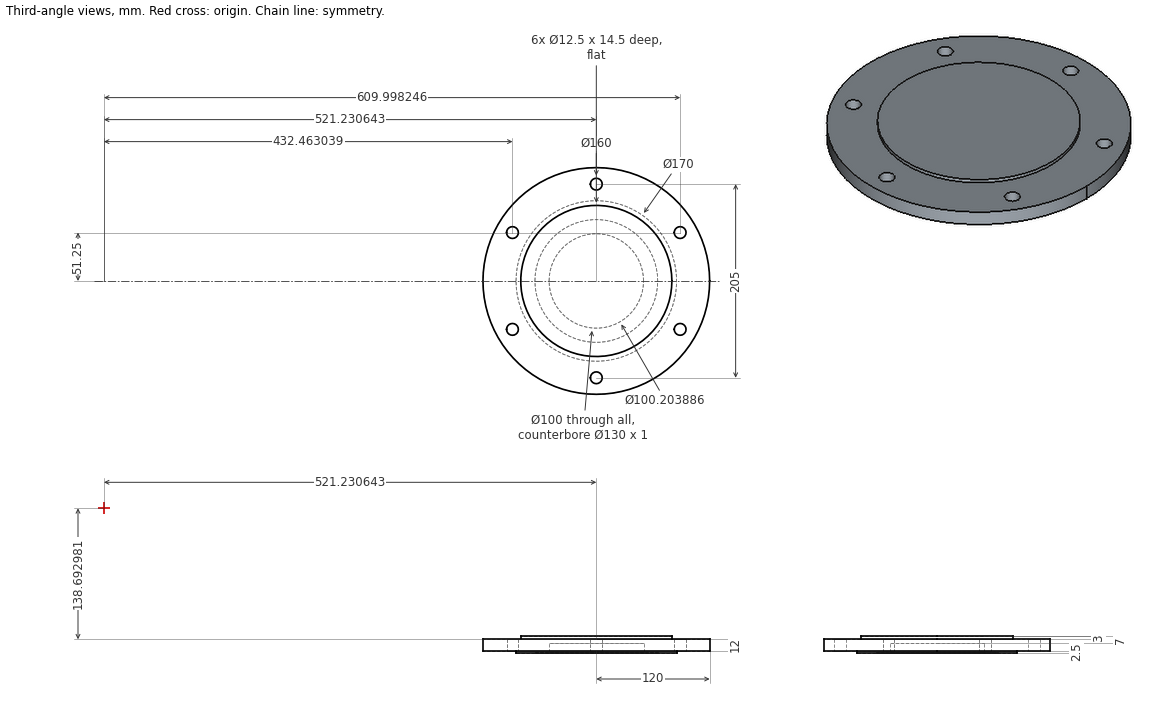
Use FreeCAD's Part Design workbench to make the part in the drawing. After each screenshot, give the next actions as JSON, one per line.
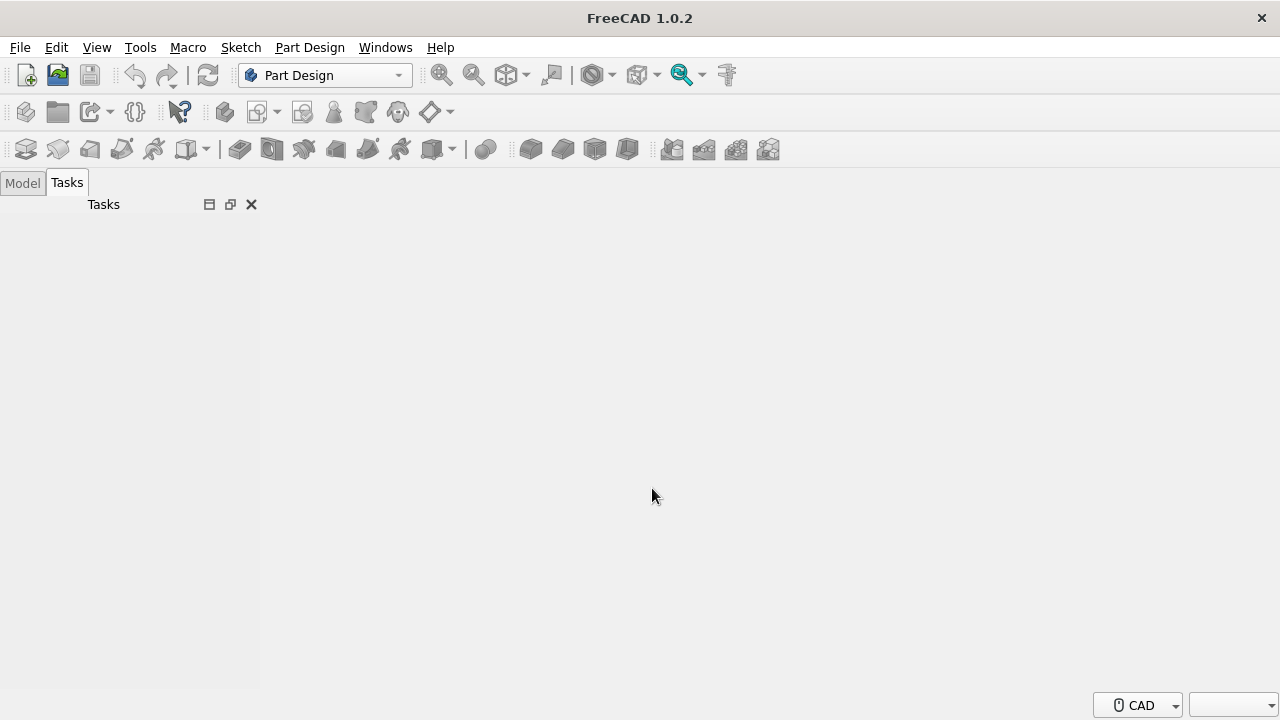
{"action": "left_click", "coordinate": [26, 76]}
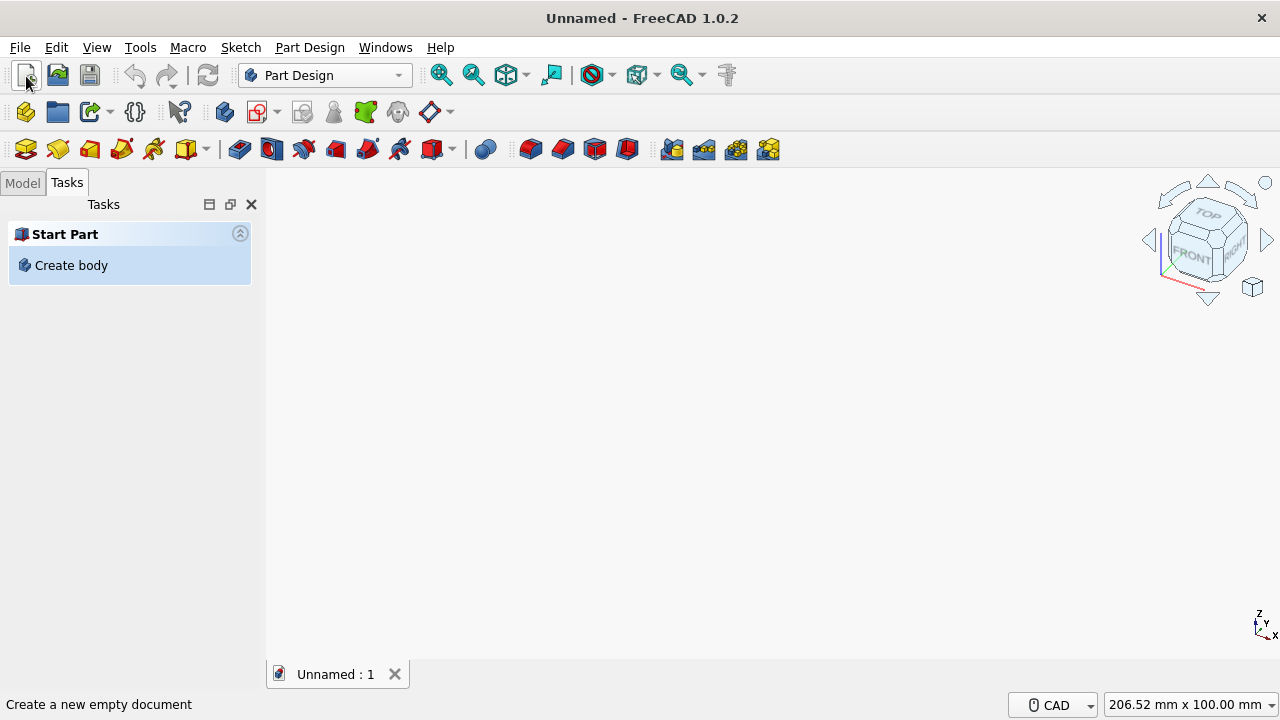
{"action": "left_click", "coordinate": [226, 112]}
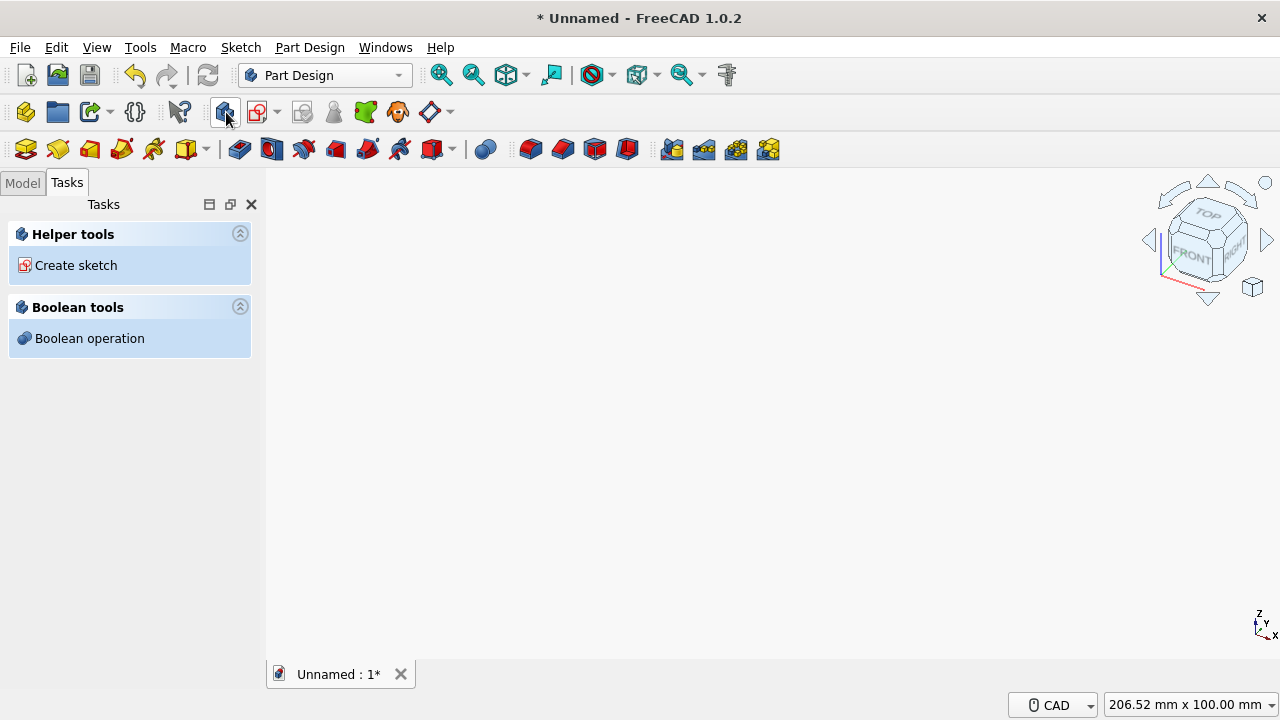
{"action": "left_click", "coordinate": [23, 182]}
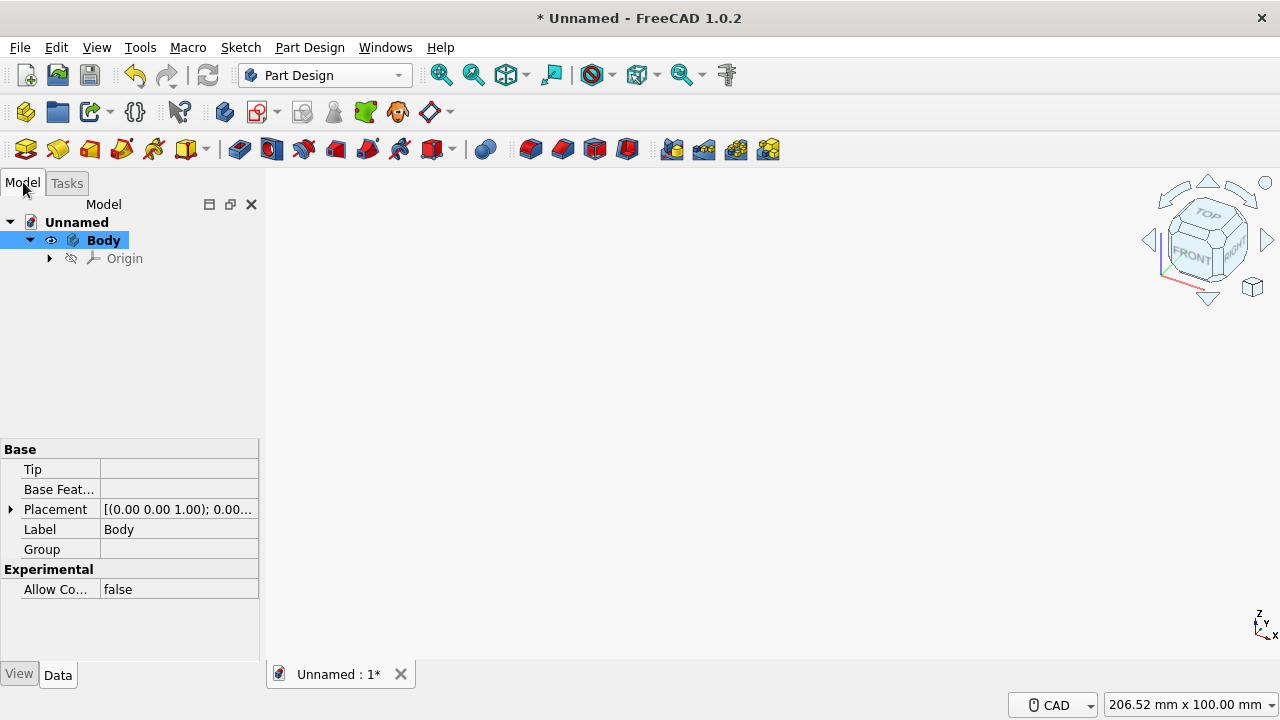
{"action": "left_click", "coordinate": [50, 258]}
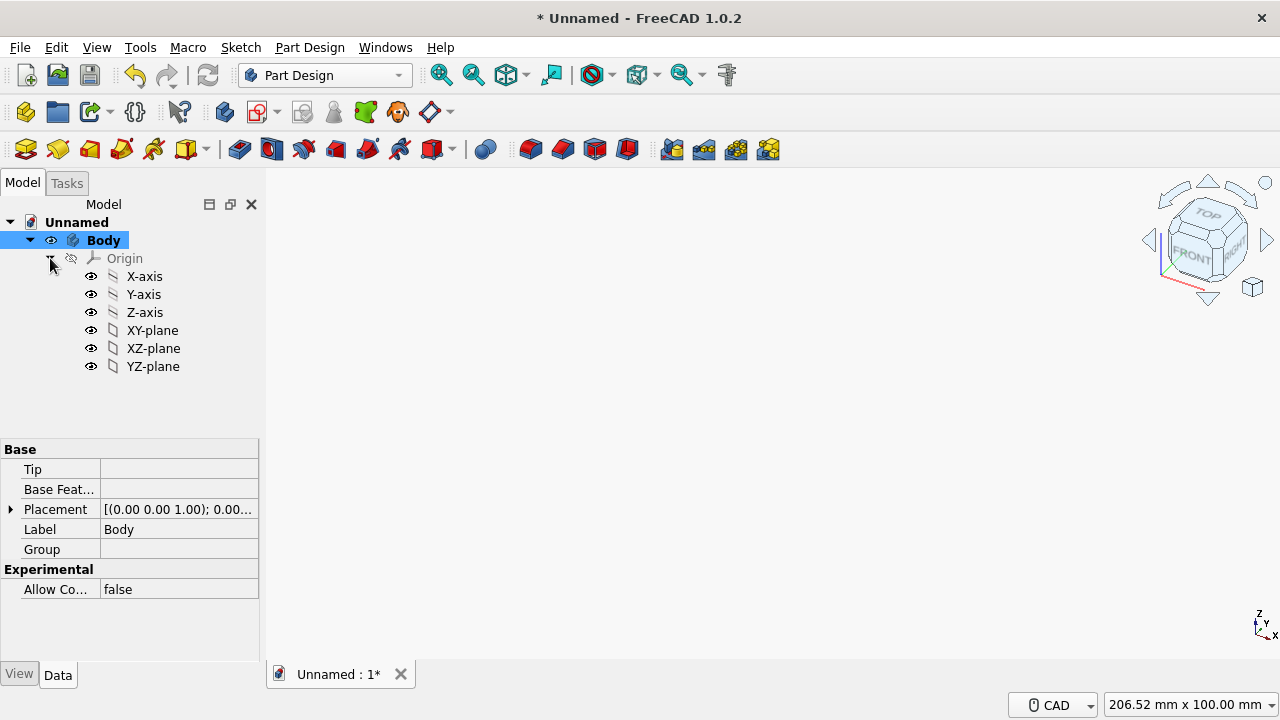
{"action": "left_click", "coordinate": [136, 348]}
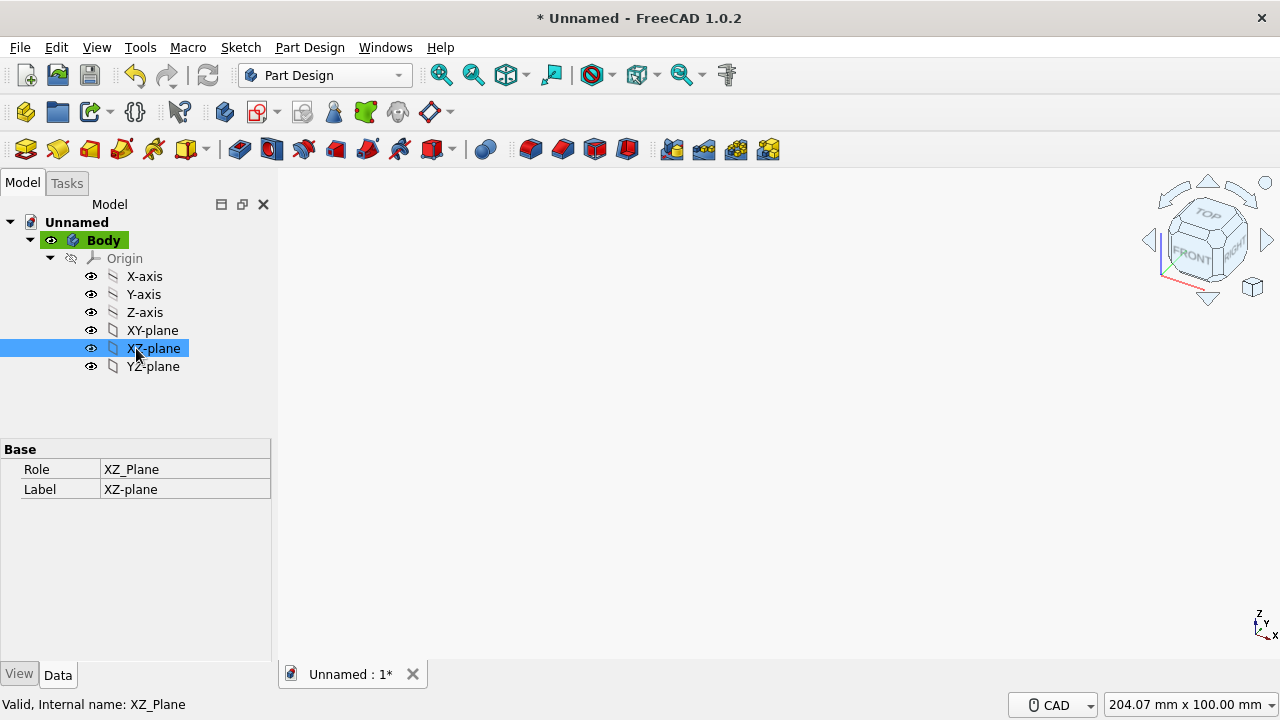
{"action": "left_click", "coordinate": [430, 112]}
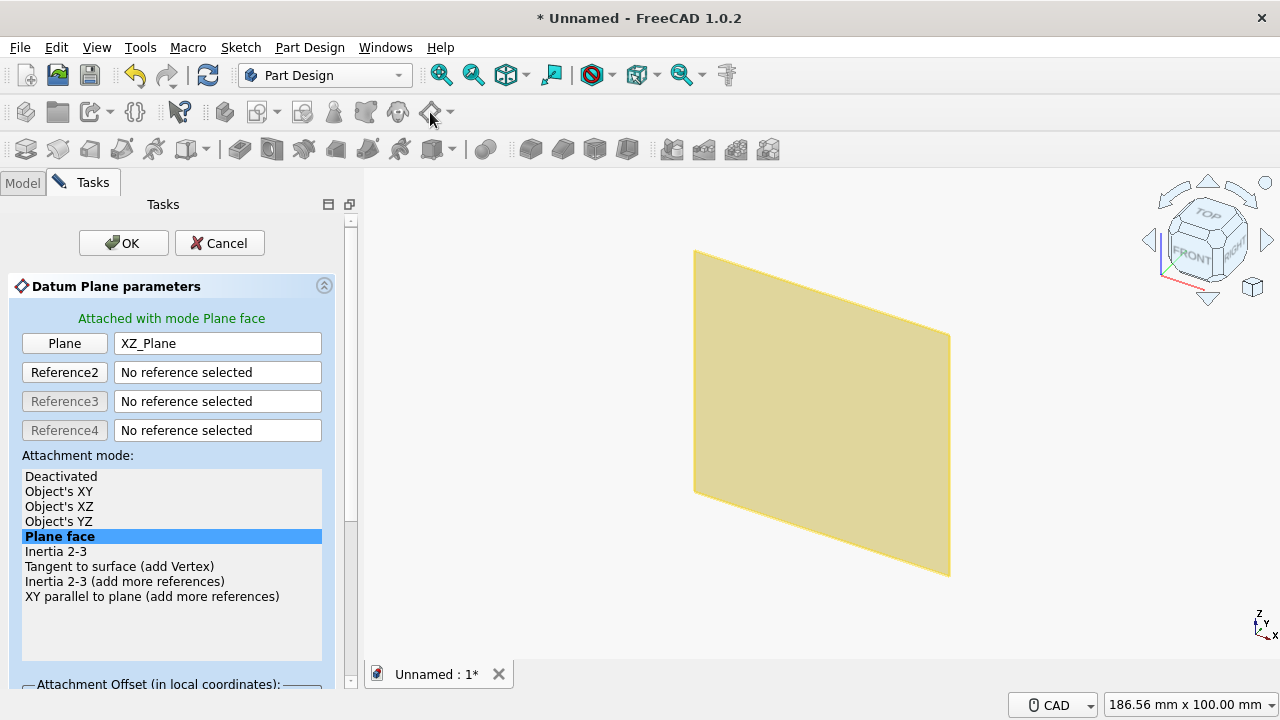
{"action": "scroll", "coordinate": [351, 451], "scroll_direction": "down", "scroll_amount": 3}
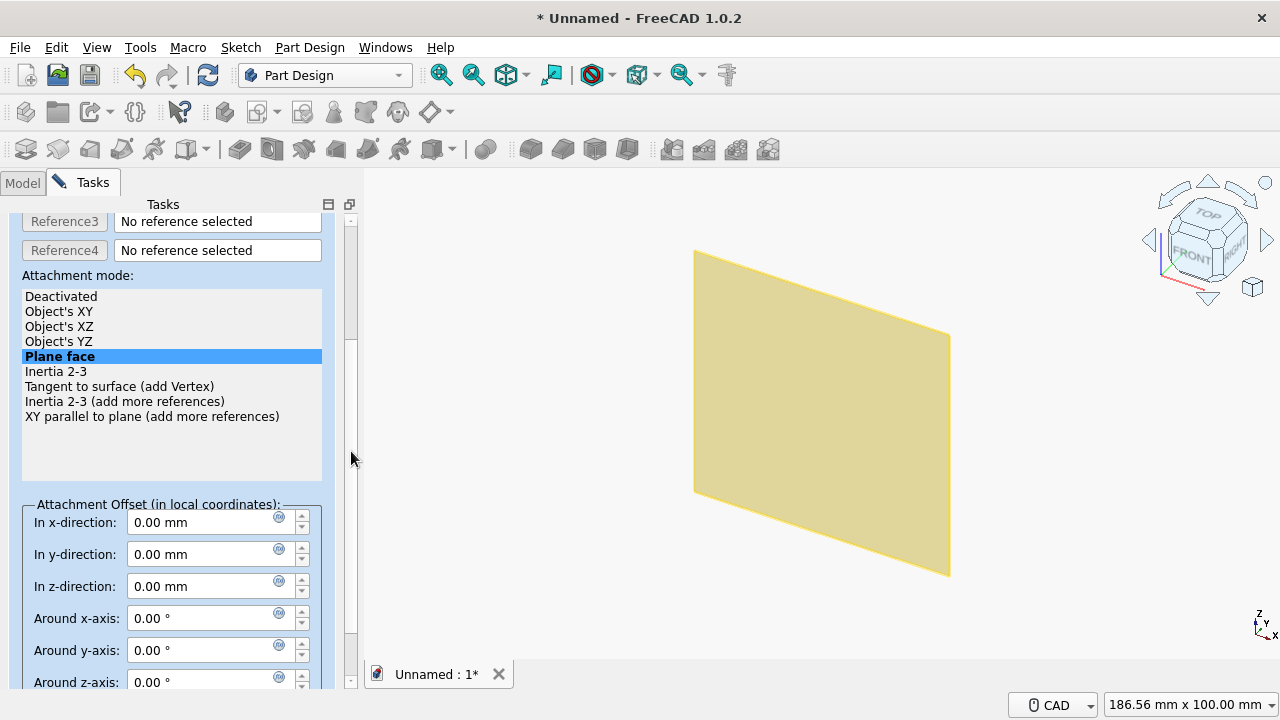
{"action": "triple_click", "coordinate": [210, 586]}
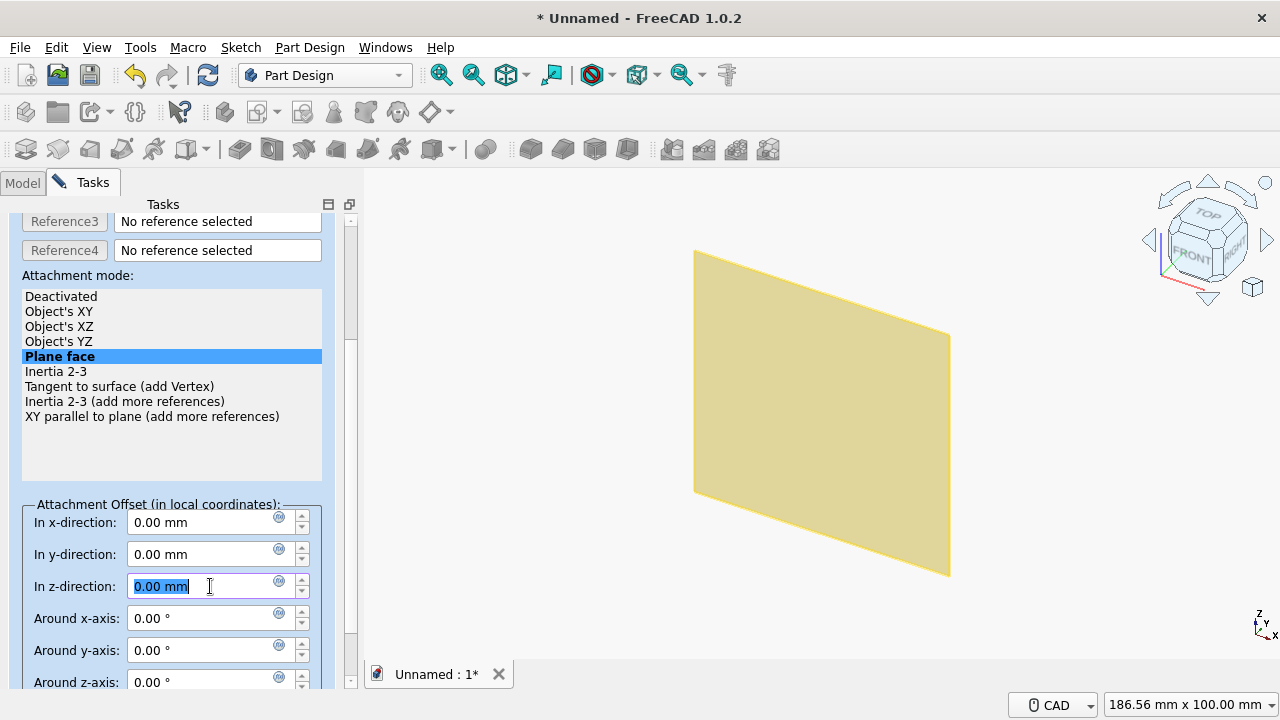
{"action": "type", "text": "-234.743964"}
{"action": "key", "text": "Tab"}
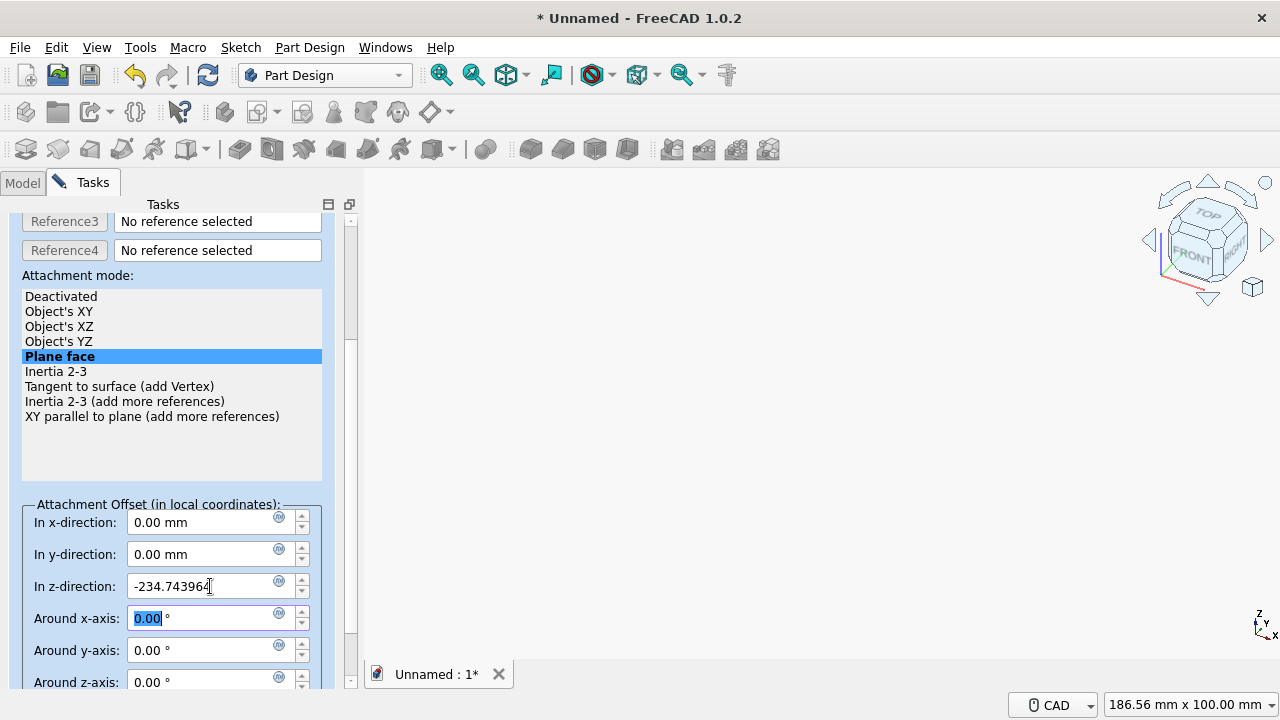
{"action": "scroll", "coordinate": [351, 451], "scroll_direction": "up", "scroll_amount": 4}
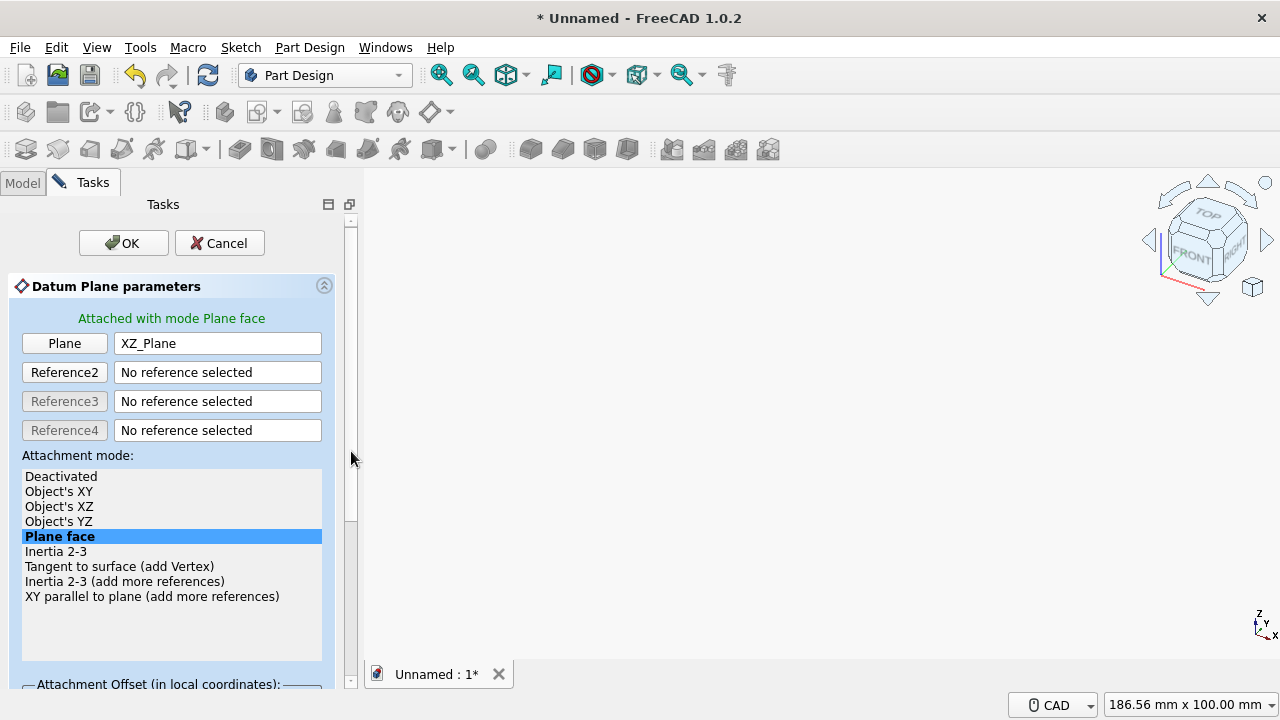
{"action": "left_click", "coordinate": [124, 243]}